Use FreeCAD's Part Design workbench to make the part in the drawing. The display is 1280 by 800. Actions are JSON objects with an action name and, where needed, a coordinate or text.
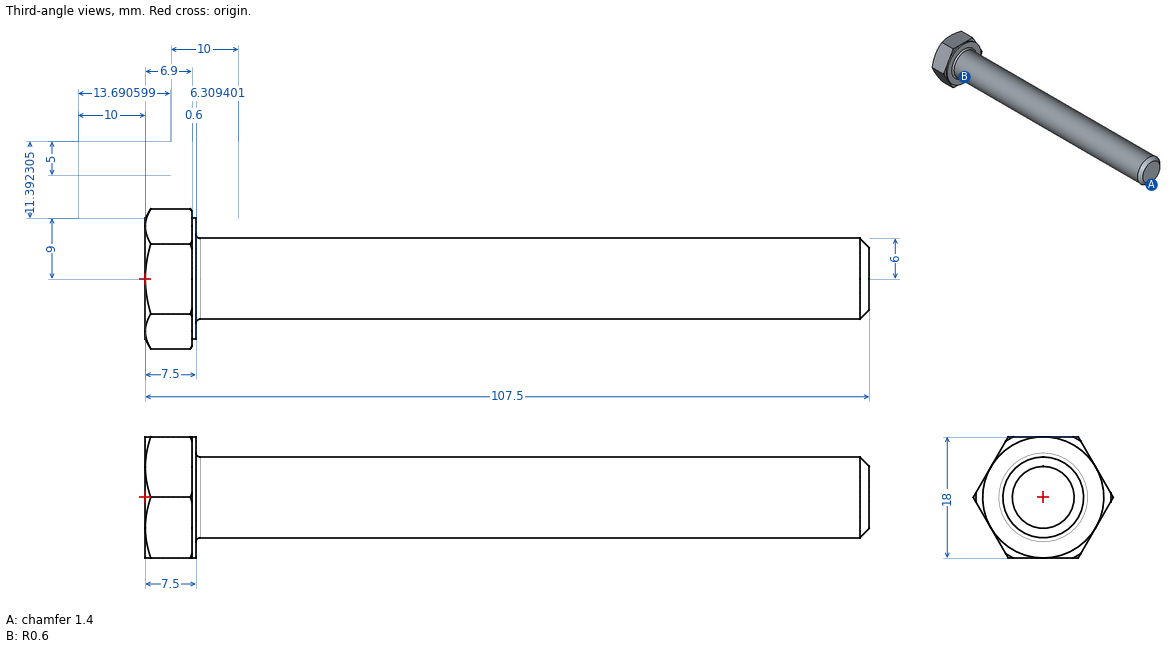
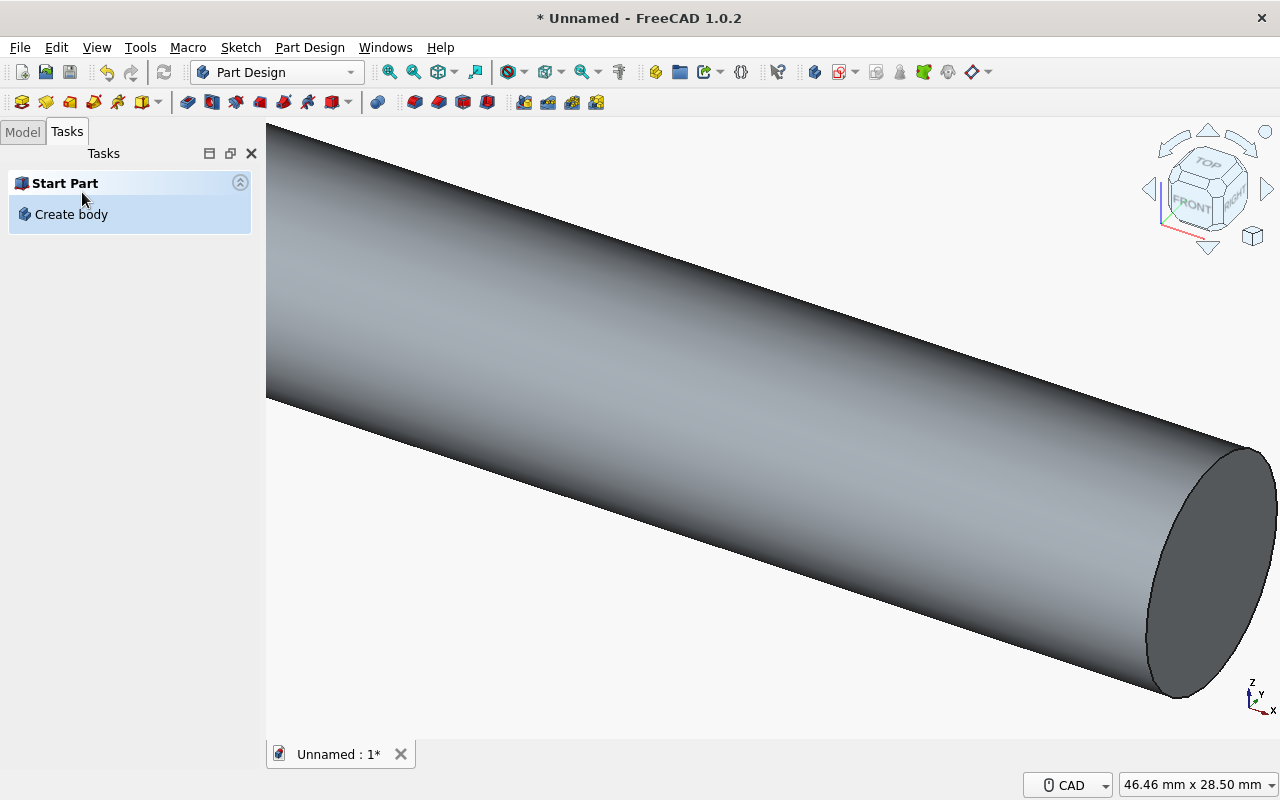
{"action": "left_click", "coordinate": [390, 72]}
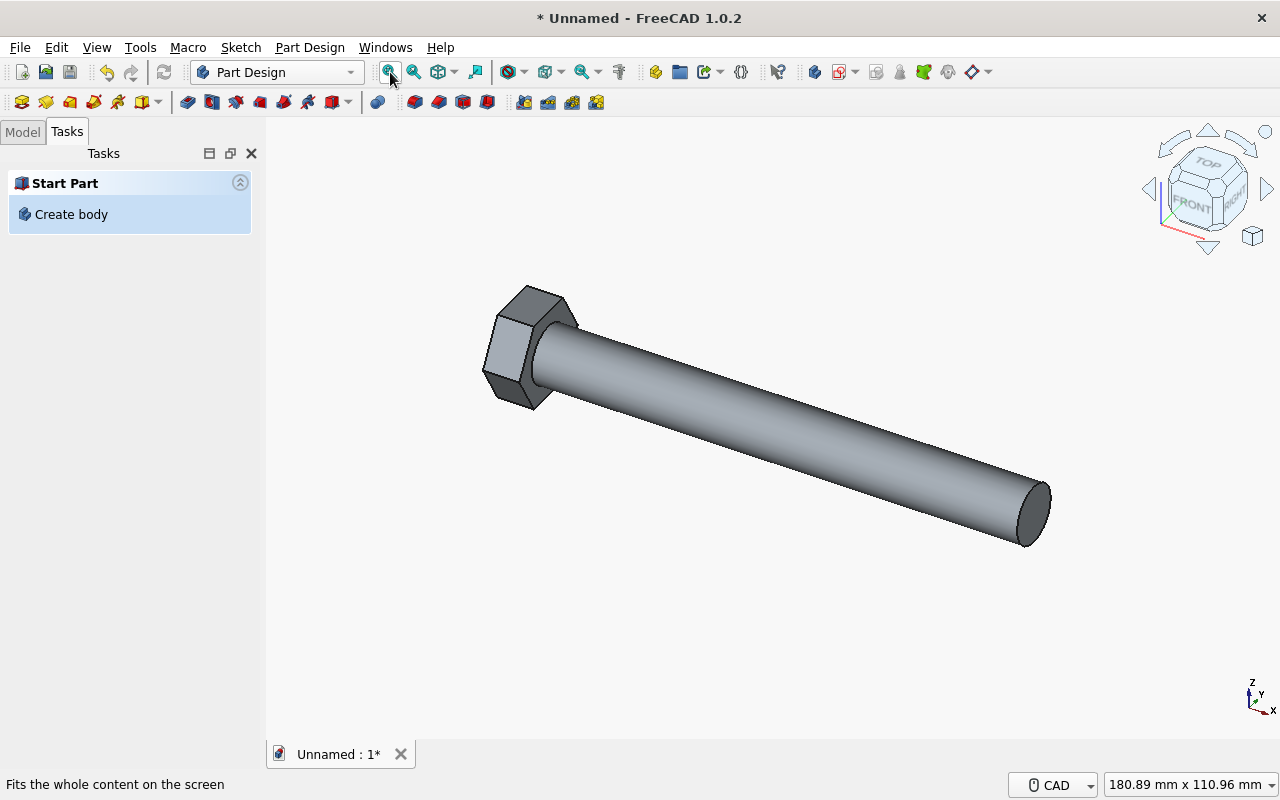
{"action": "left_click", "coordinate": [840, 72]}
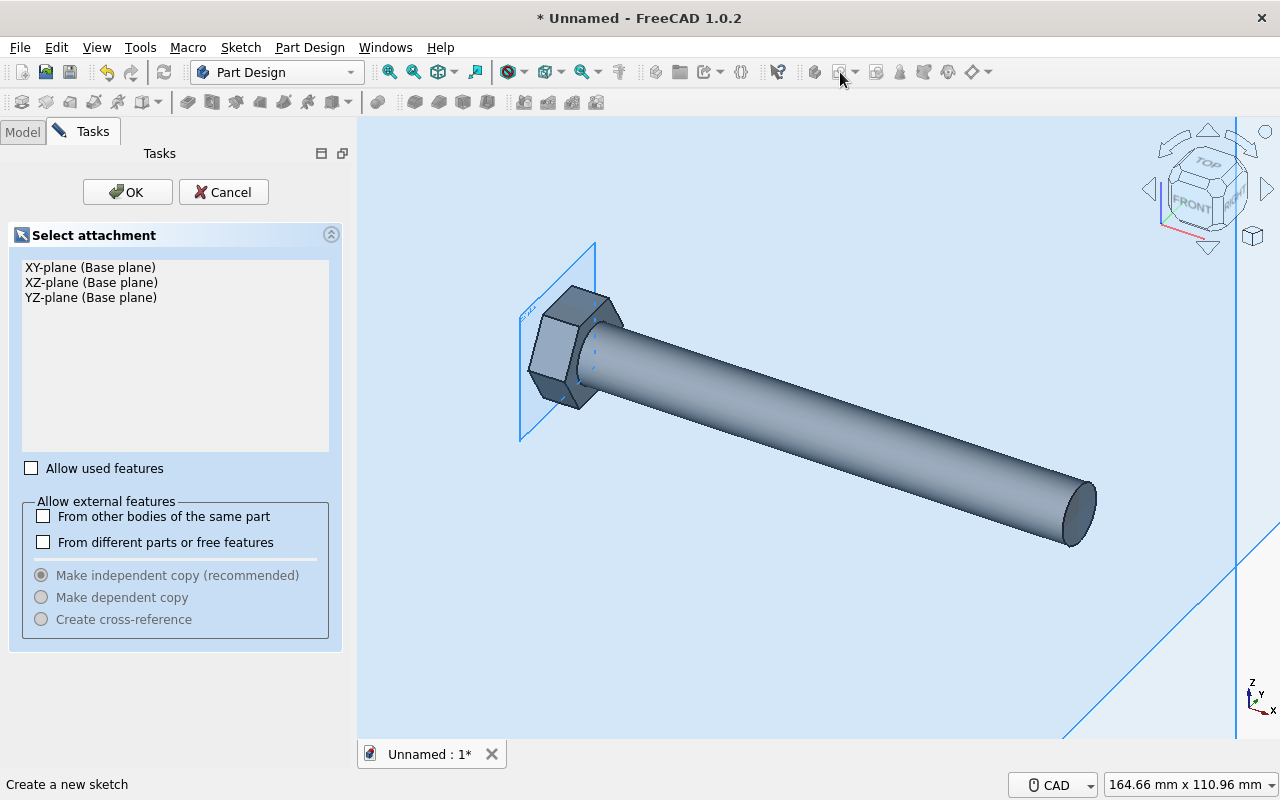
{"action": "left_click", "coordinate": [82, 268]}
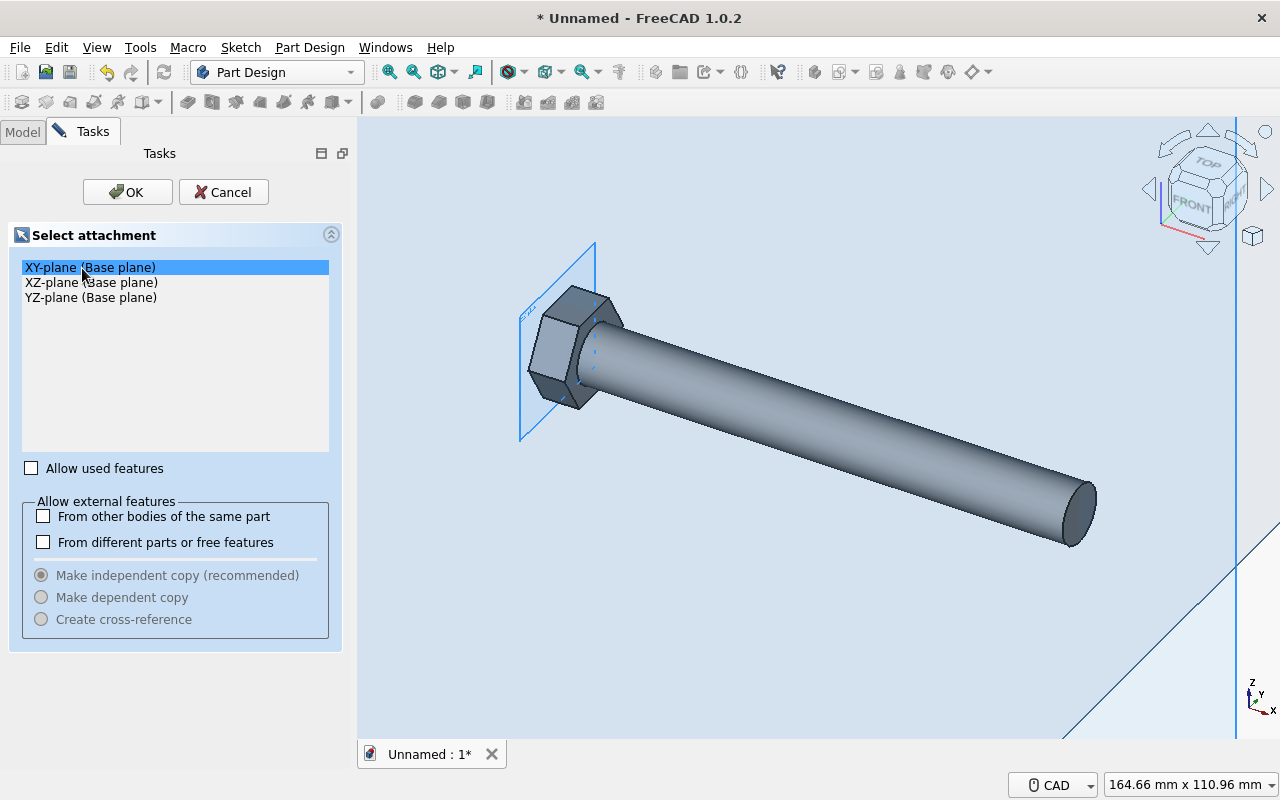
{"action": "left_click", "coordinate": [128, 192]}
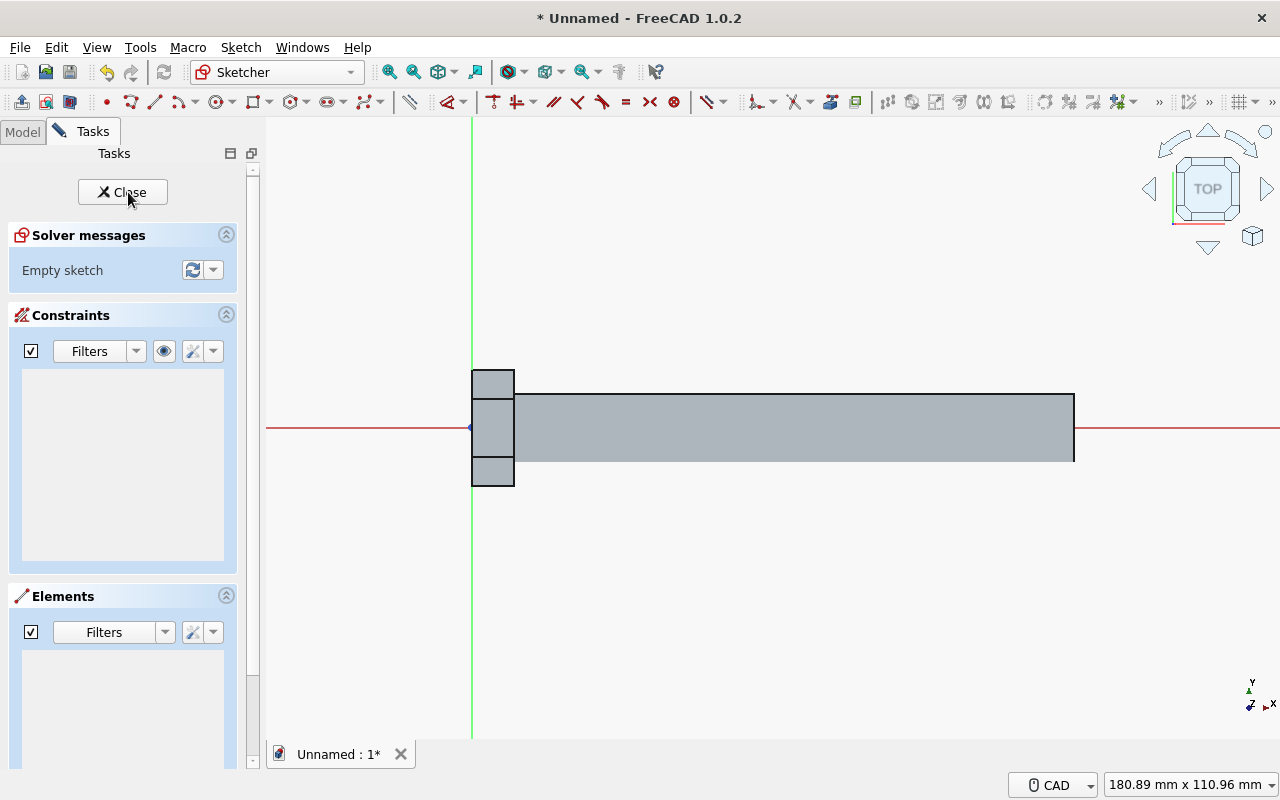
{"action": "key", "text": "q s"}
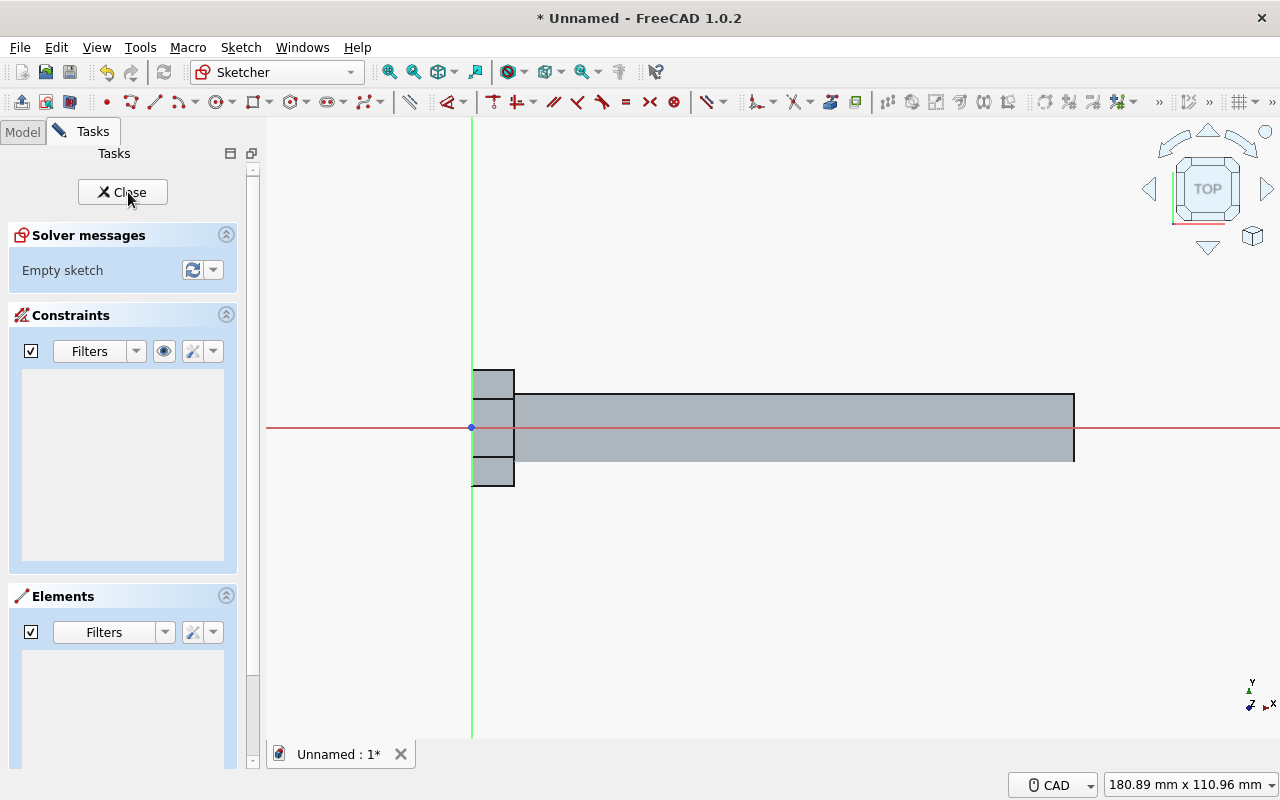
{"action": "scroll", "coordinate": [346, 346], "scroll_direction": "up", "scroll_amount": 6}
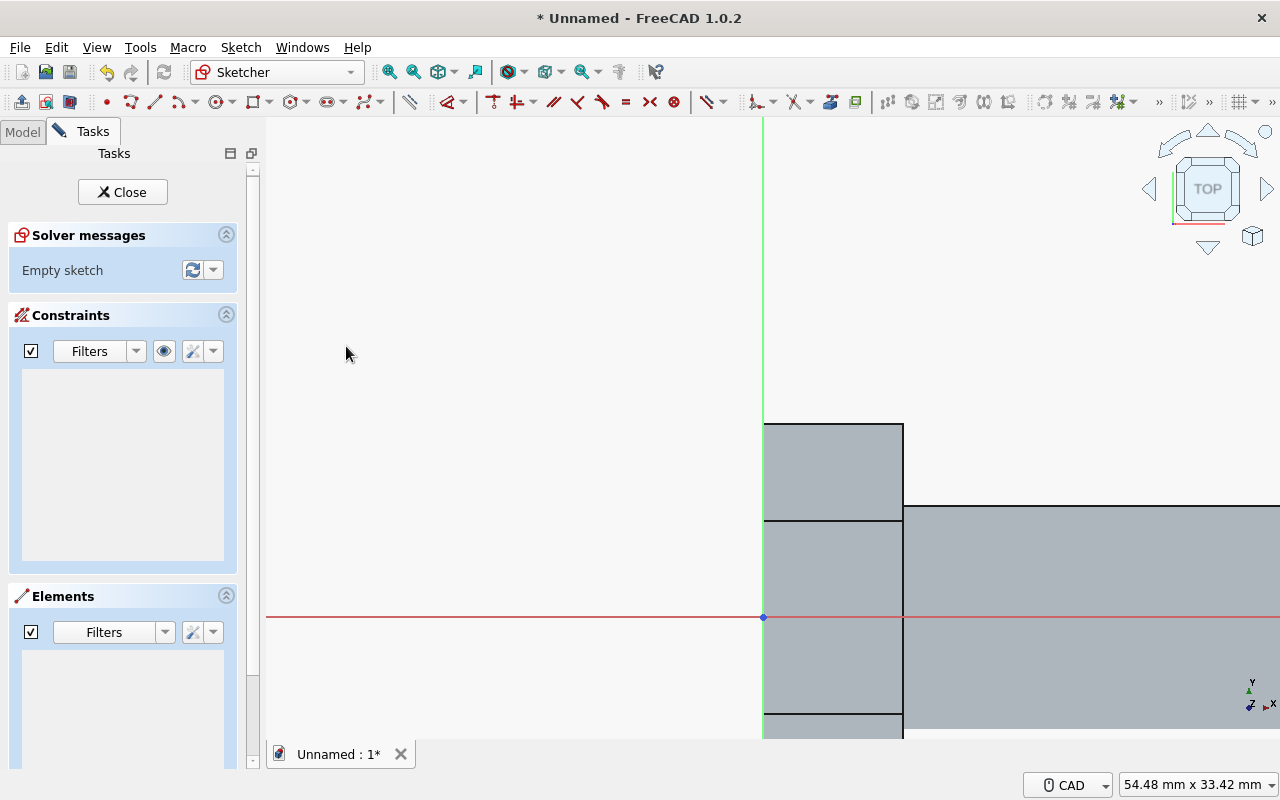
{"action": "key", "text": "g m"}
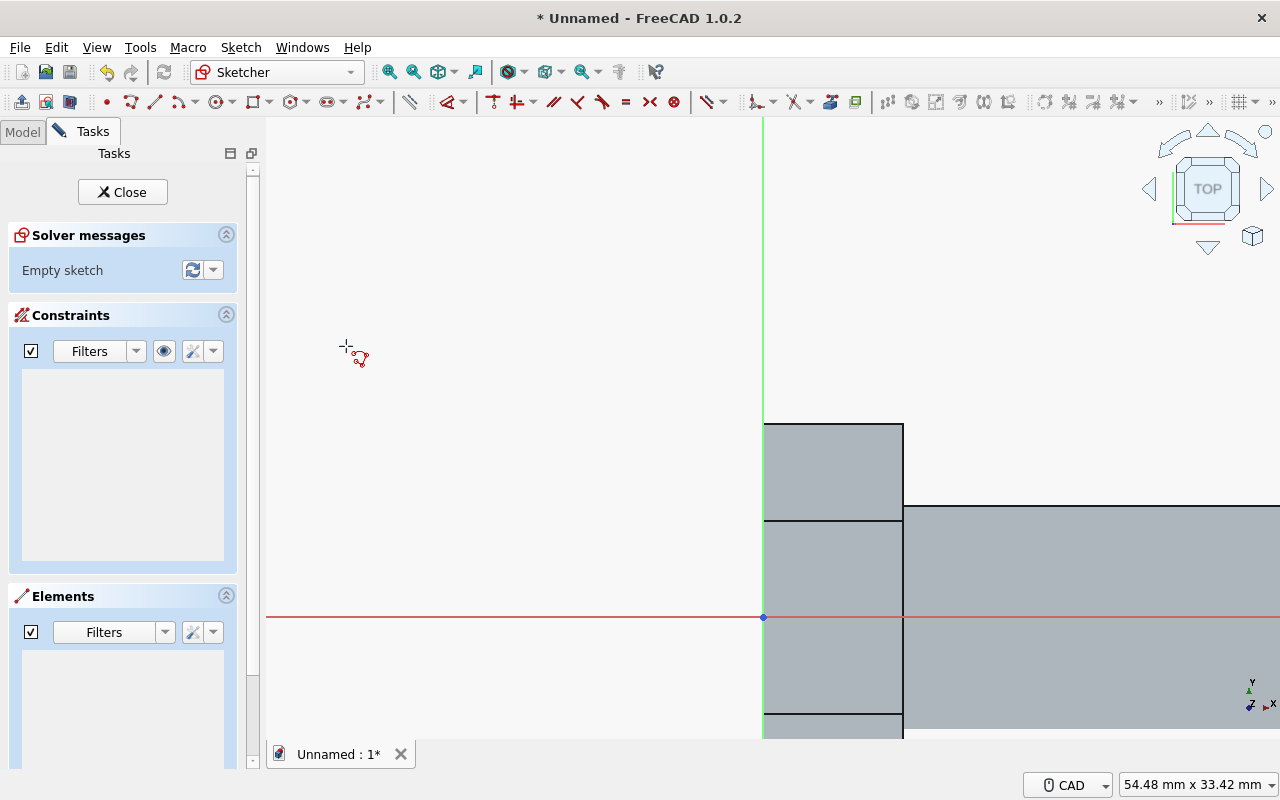
{"action": "left_click", "coordinate": [763, 450]}
{"action": "left_click", "coordinate": [832, 331]}
{"action": "left_click", "coordinate": [832, 238]}
{"action": "left_click", "coordinate": [577, 238]}
{"action": "left_click", "coordinate": [577, 450]}
{"action": "left_click", "coordinate": [763, 451]}
{"action": "key", "text": "Escape"}
{"action": "key", "text": "Escape"}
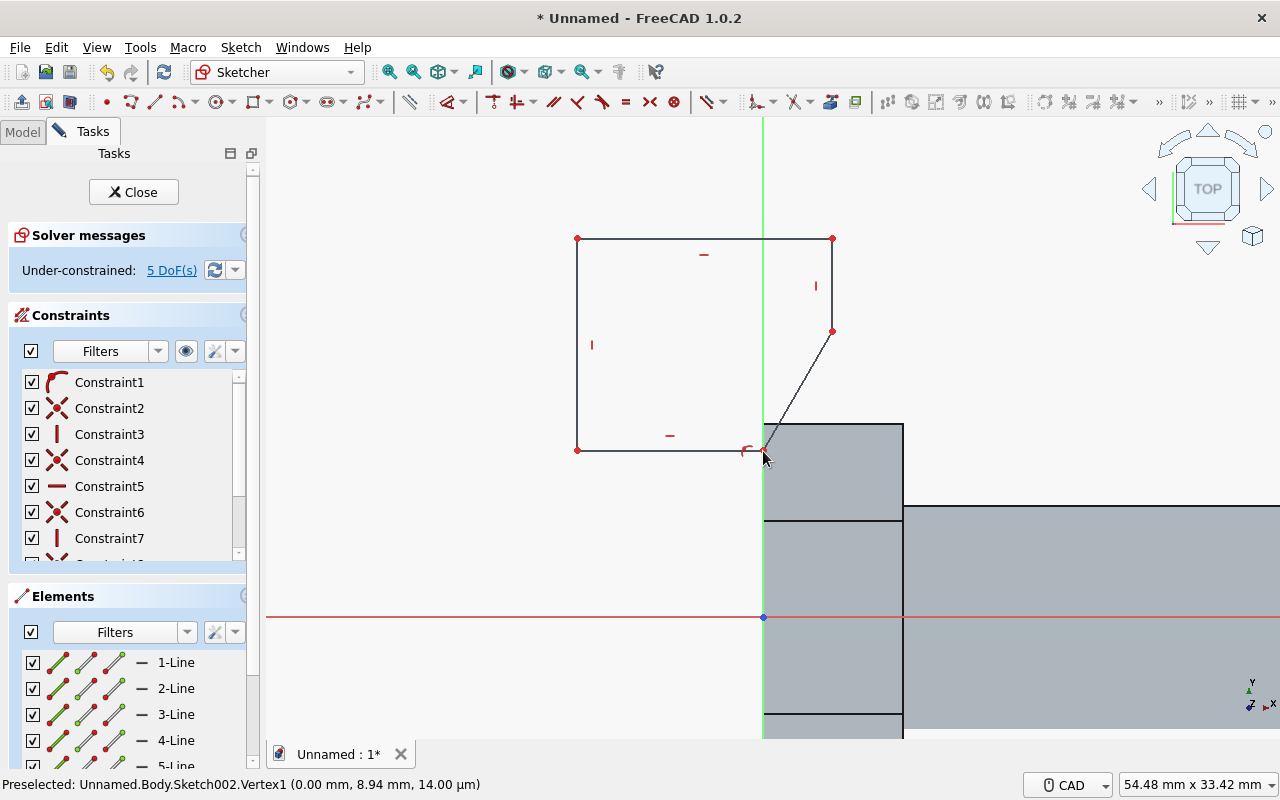
{"action": "left_click", "coordinate": [448, 102]}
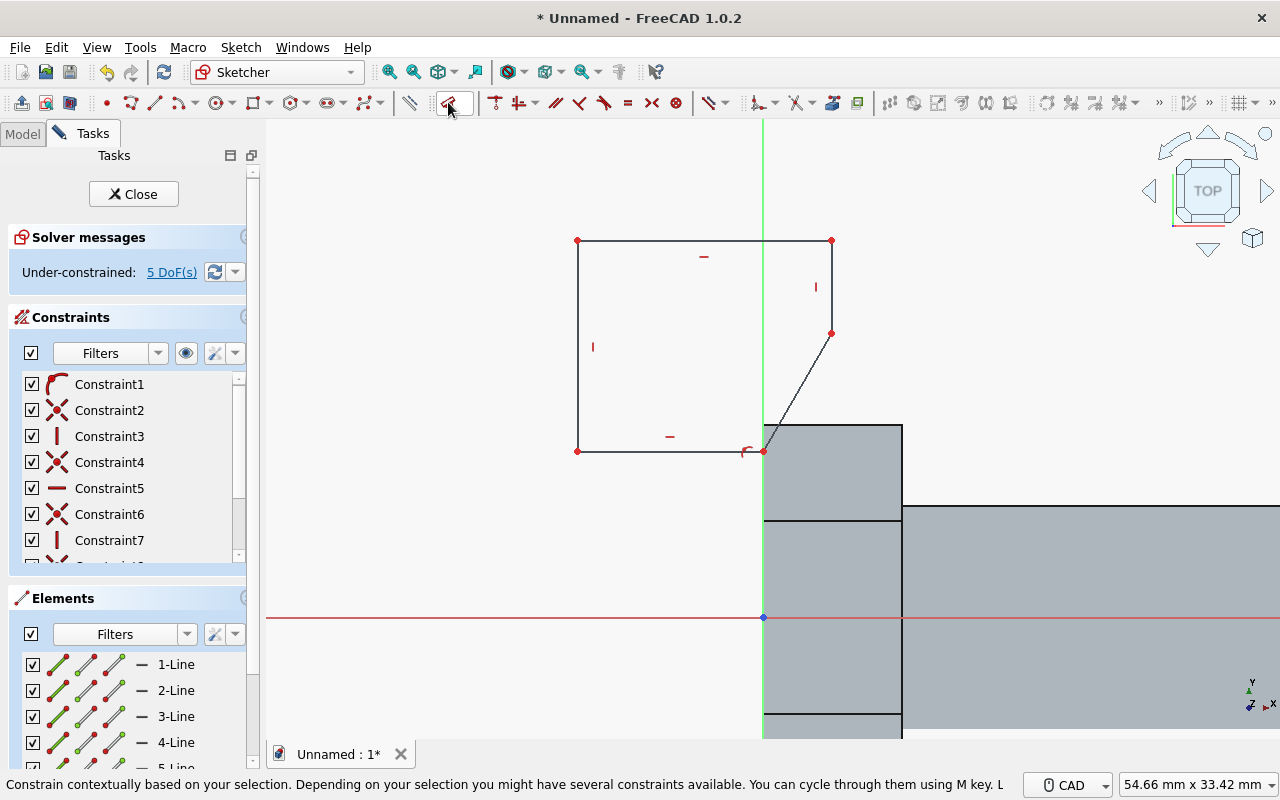
{"action": "left_click", "coordinate": [832, 305]}
{"action": "left_click", "coordinate": [866, 287]}